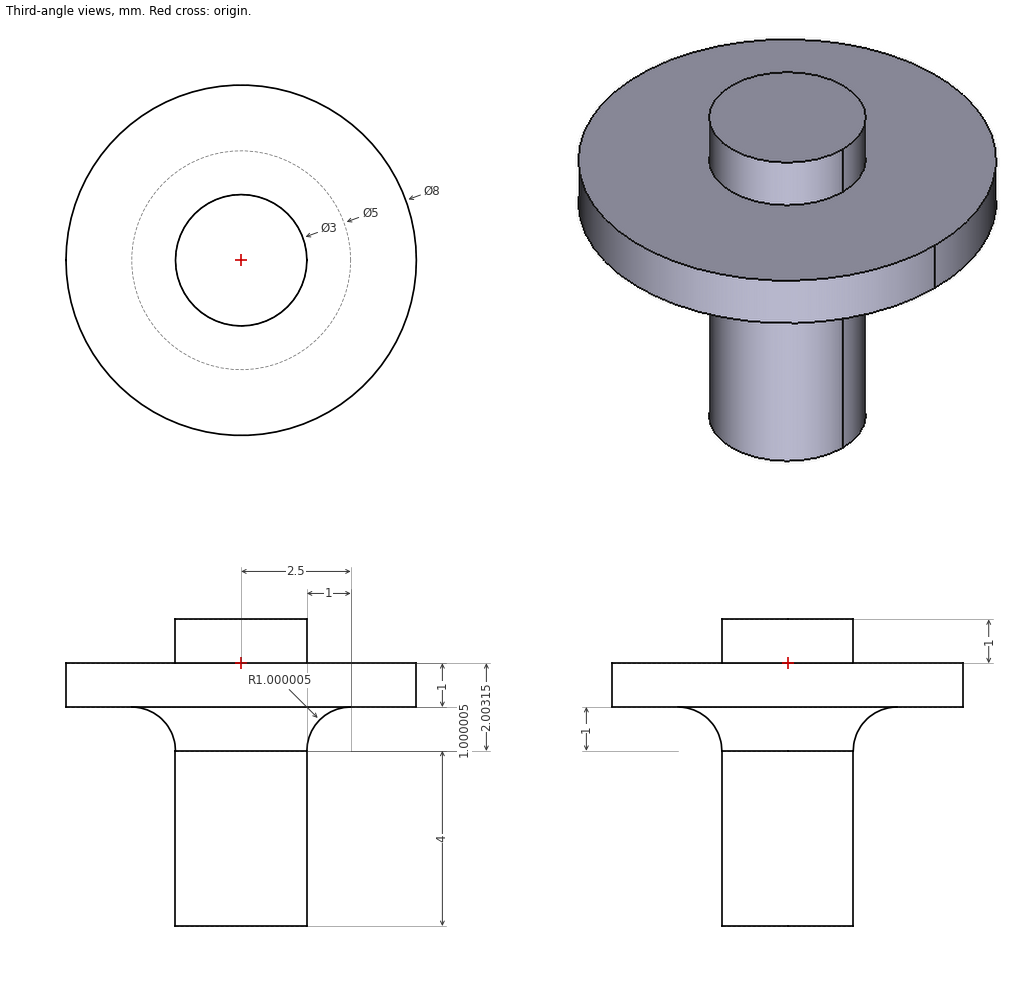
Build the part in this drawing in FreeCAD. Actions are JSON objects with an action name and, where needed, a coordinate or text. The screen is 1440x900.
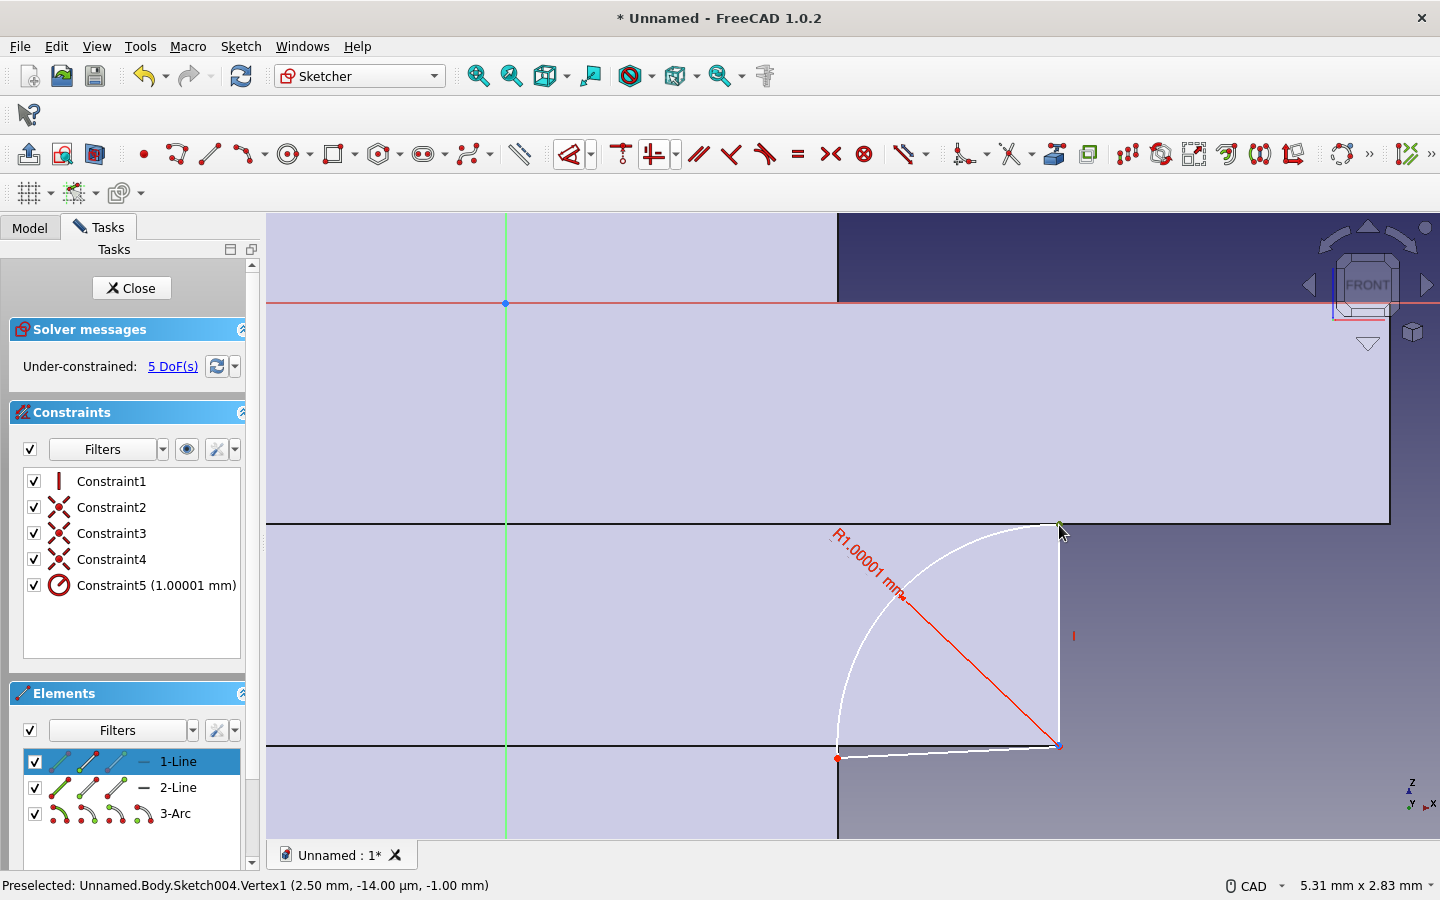
{"action": "key", "text": "i"}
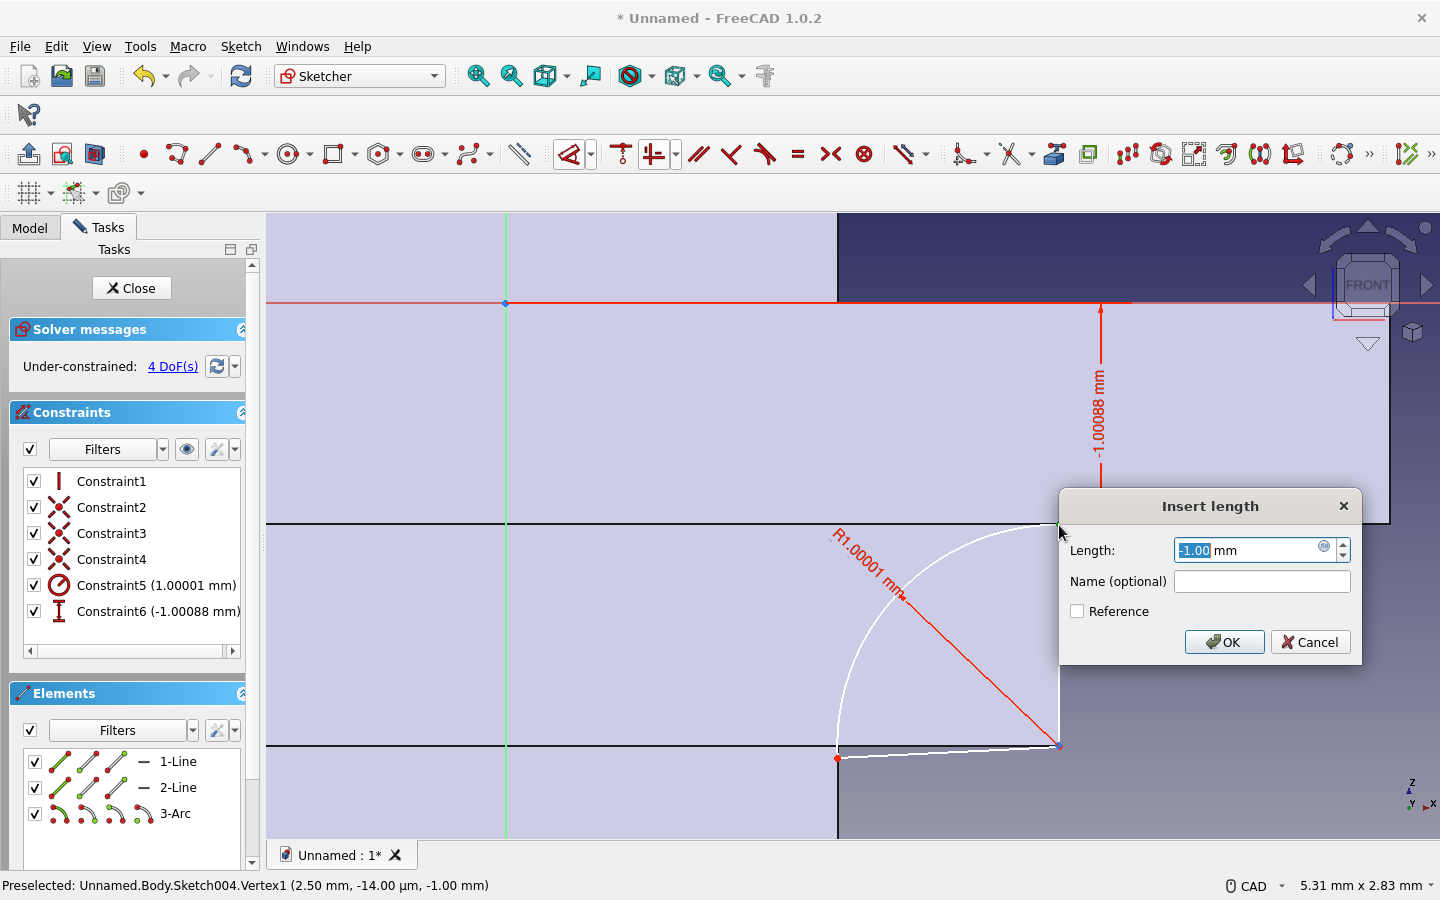
{"action": "type", "text": "-1"}
{"action": "key", "text": "Return"}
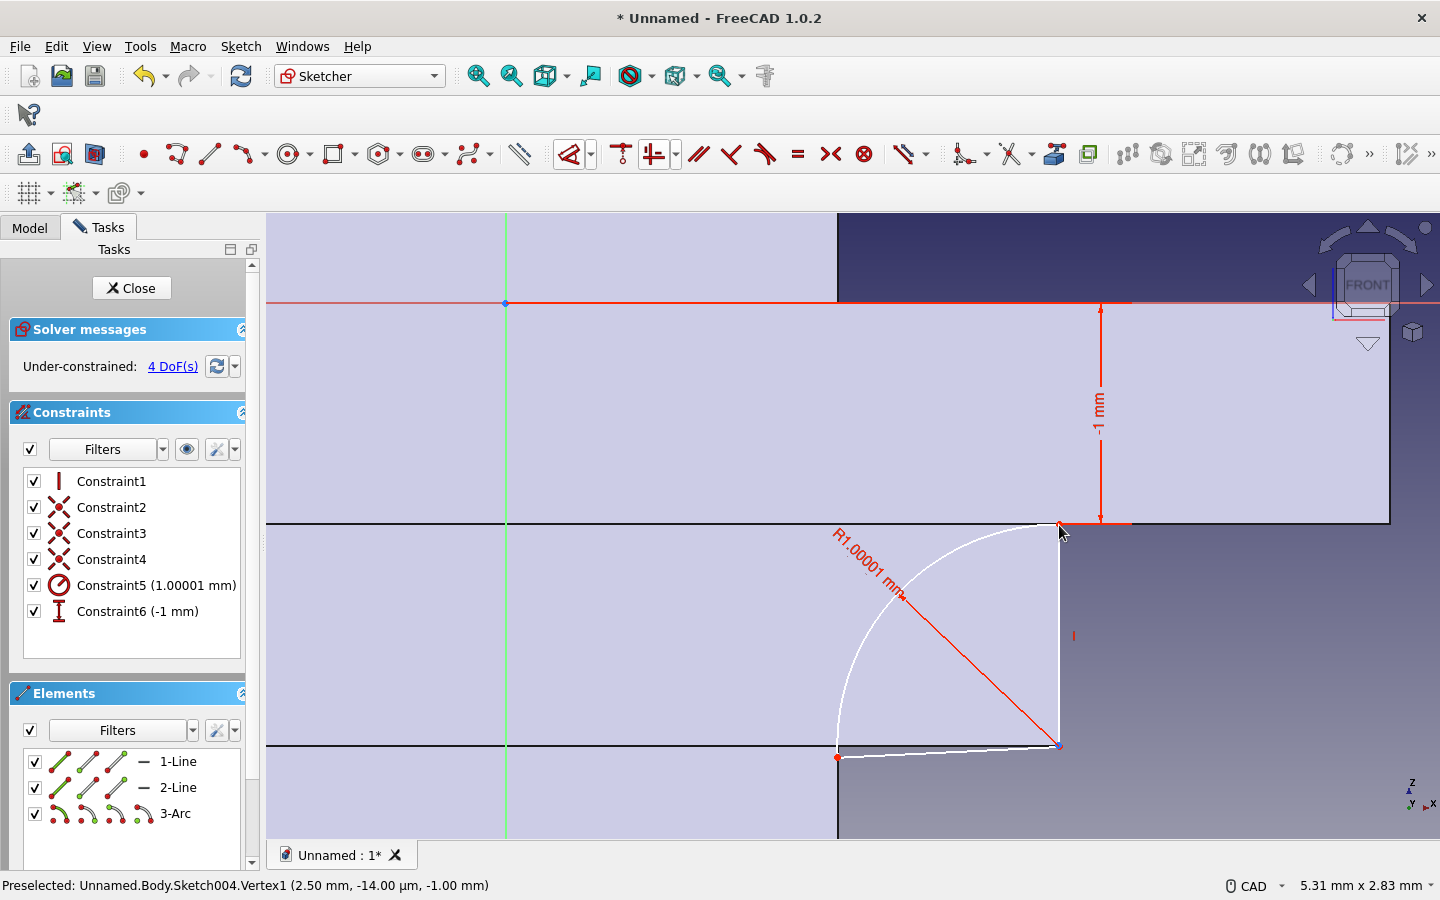
{"action": "left_click", "coordinate": [993, 750]}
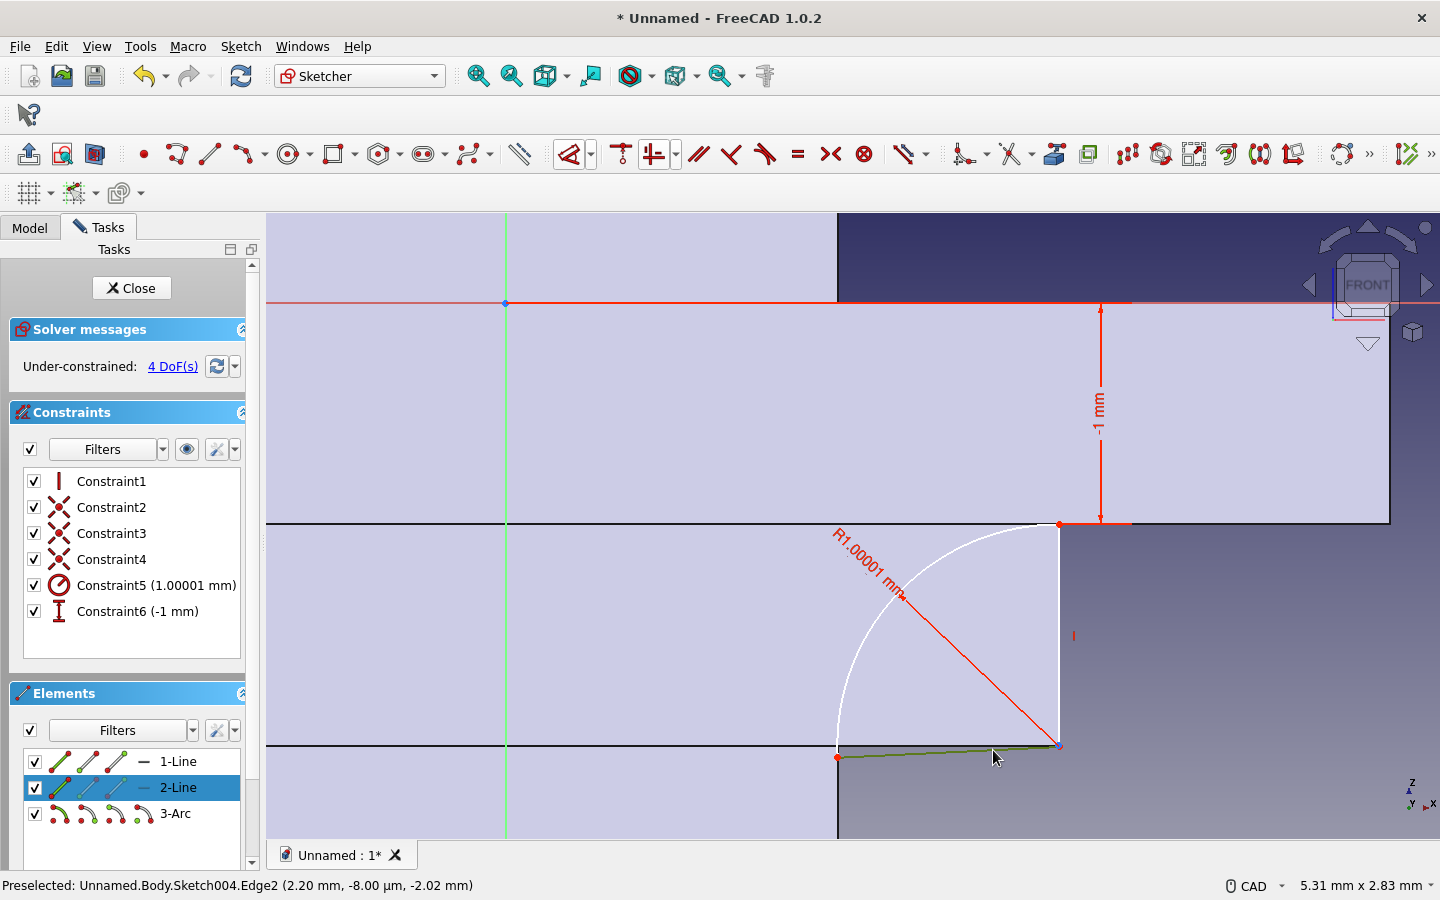
{"action": "left_click", "coordinate": [590, 154]}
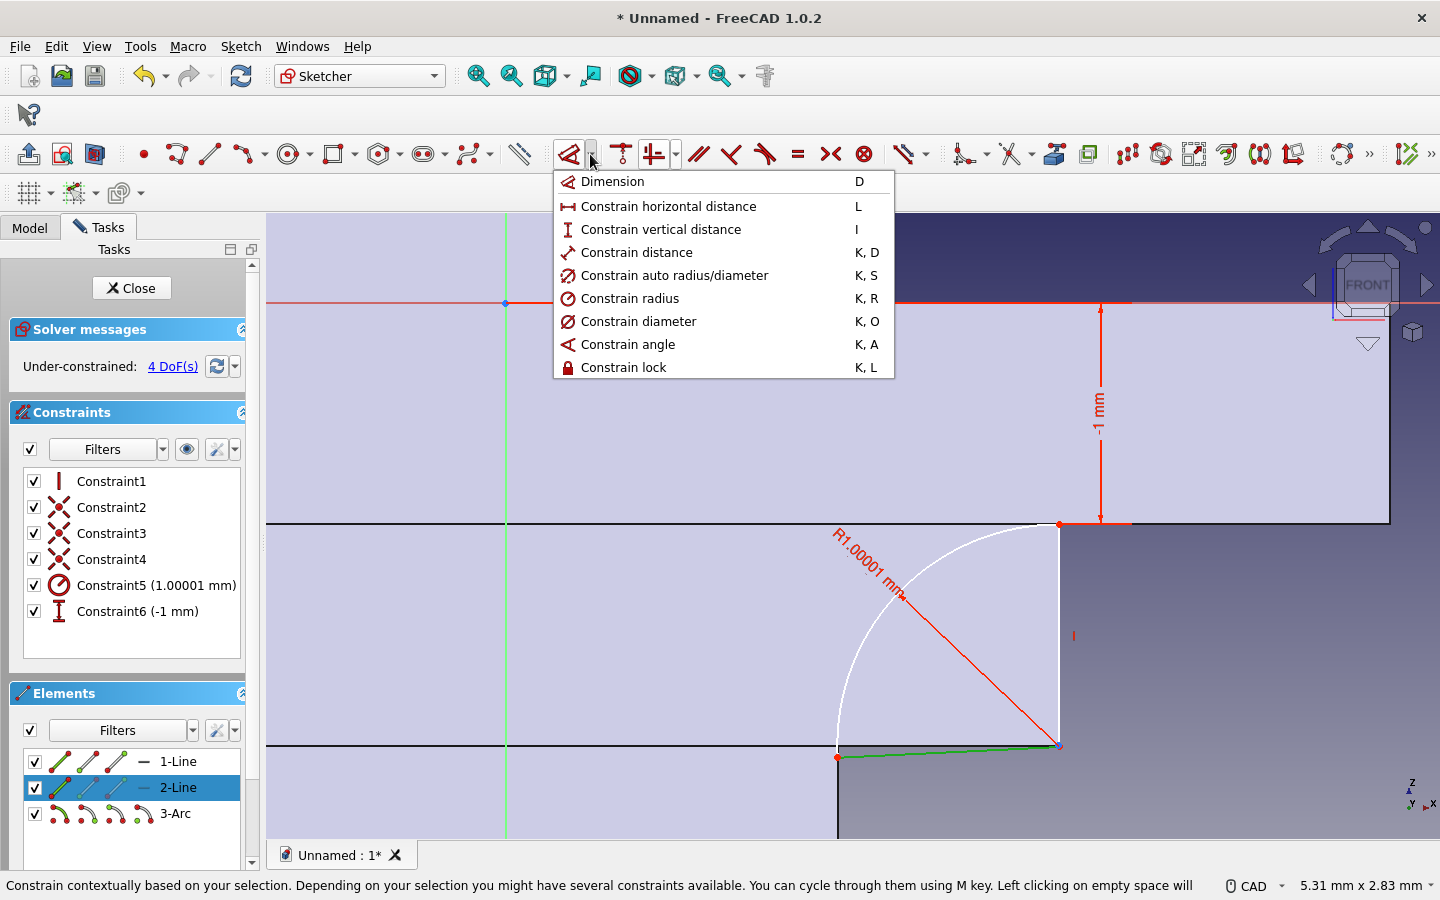
{"action": "left_click", "coordinate": [724, 206]}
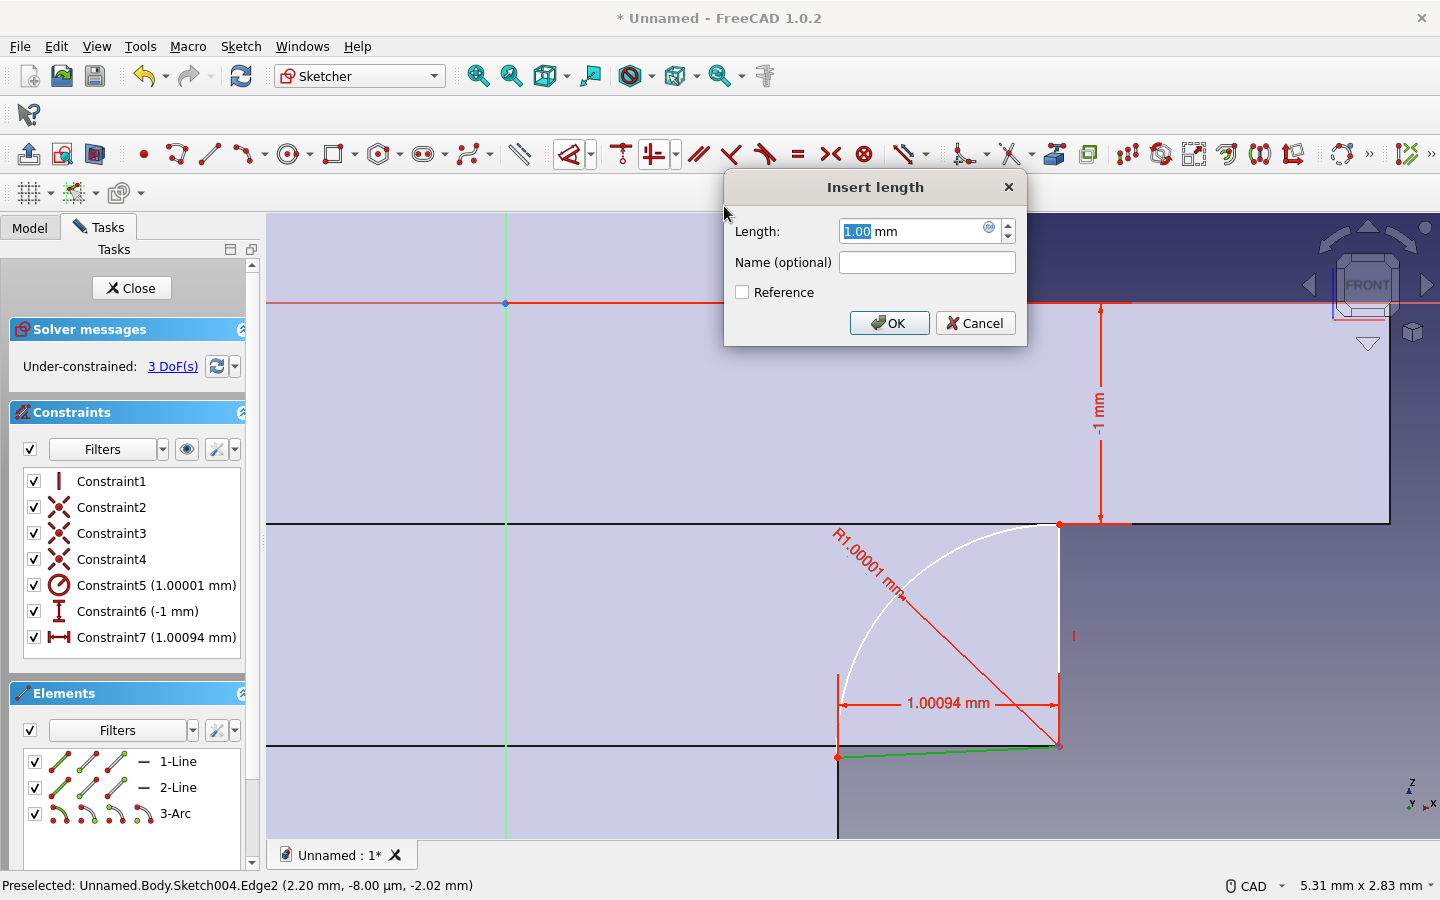
{"action": "type", "text": "1"}
{"action": "key", "text": "Return"}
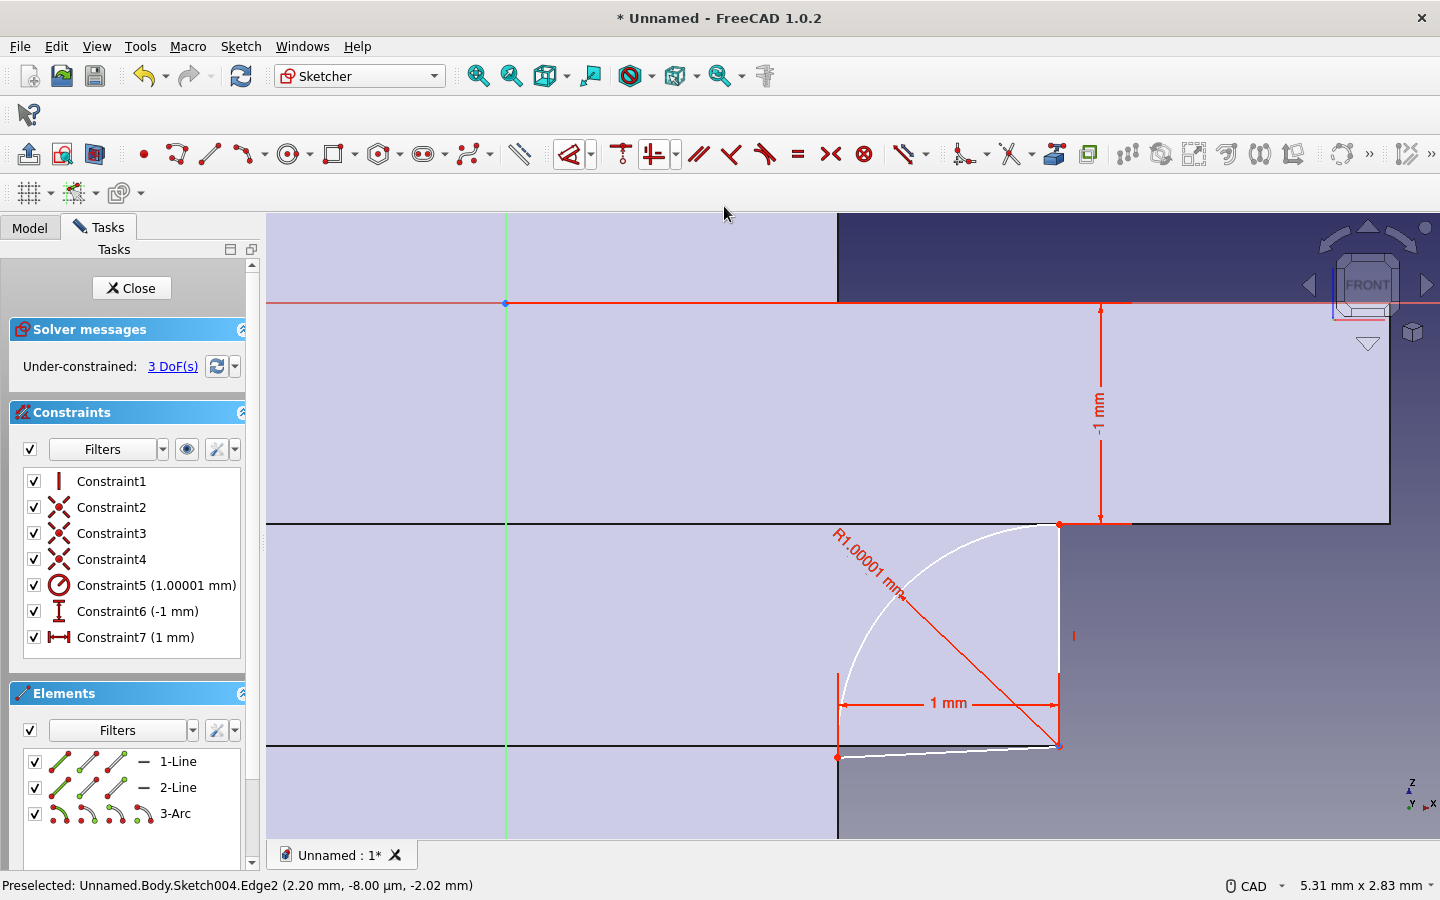
{"action": "left_click", "coordinate": [1059, 524]}